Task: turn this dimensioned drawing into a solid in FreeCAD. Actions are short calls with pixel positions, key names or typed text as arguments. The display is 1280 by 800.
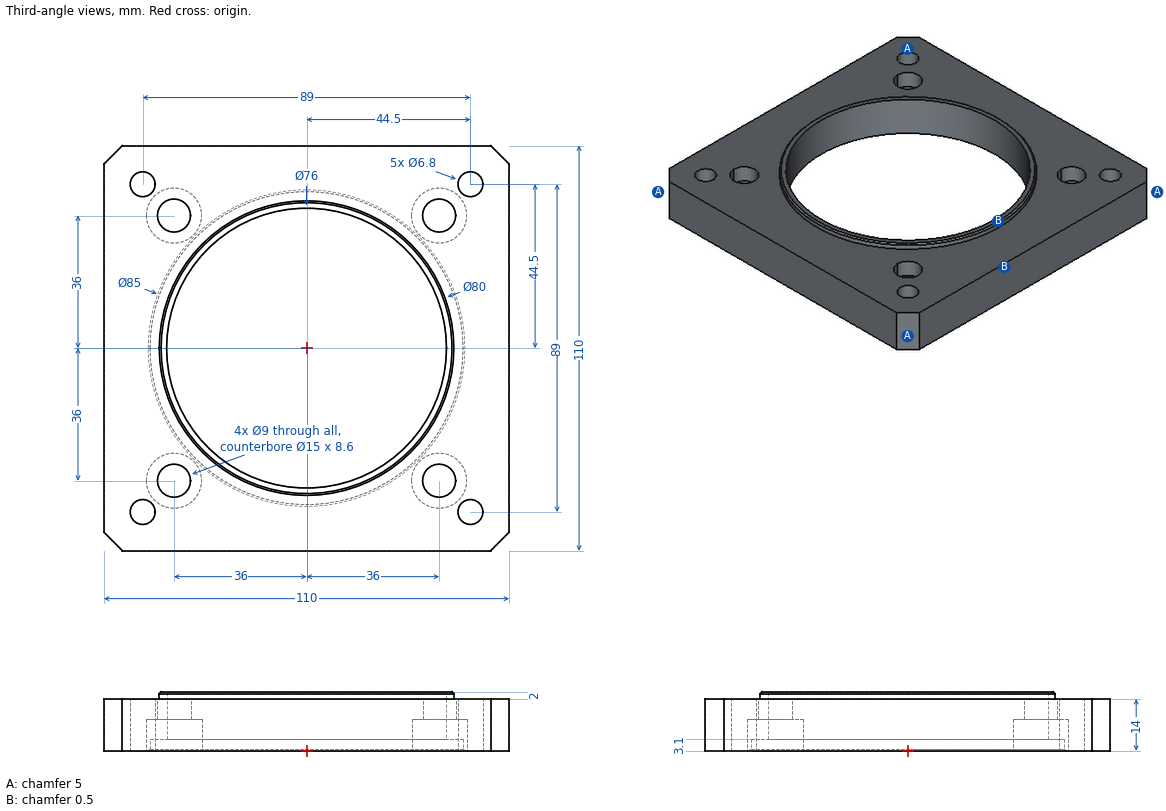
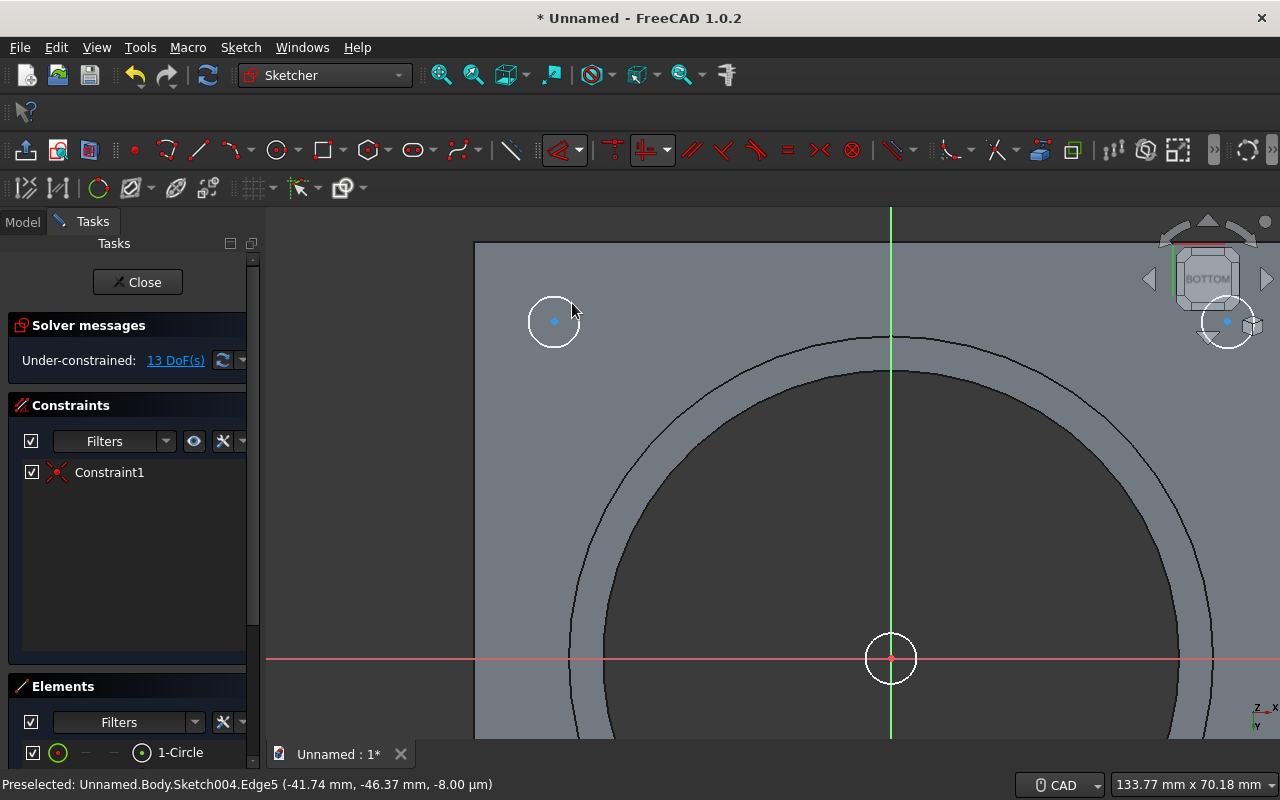
scroll(552, 322, down, 4)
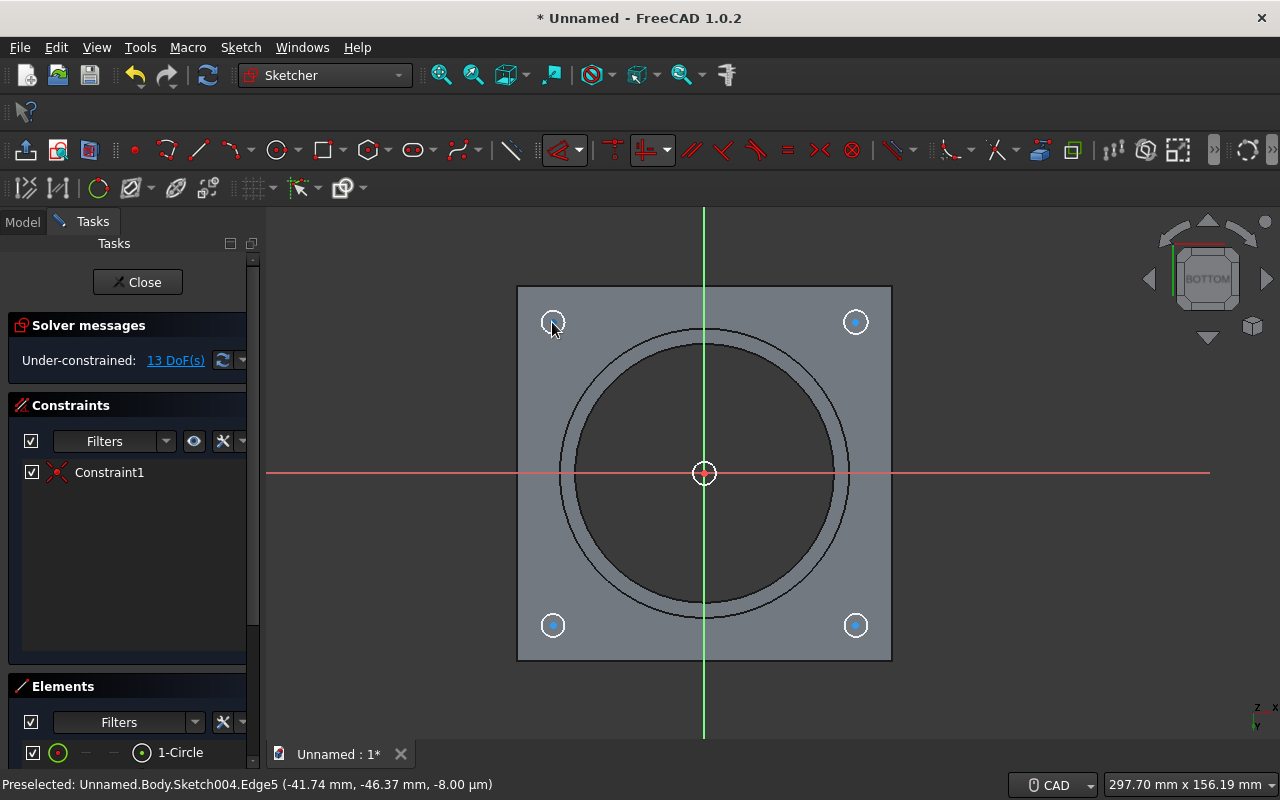
click(864, 617)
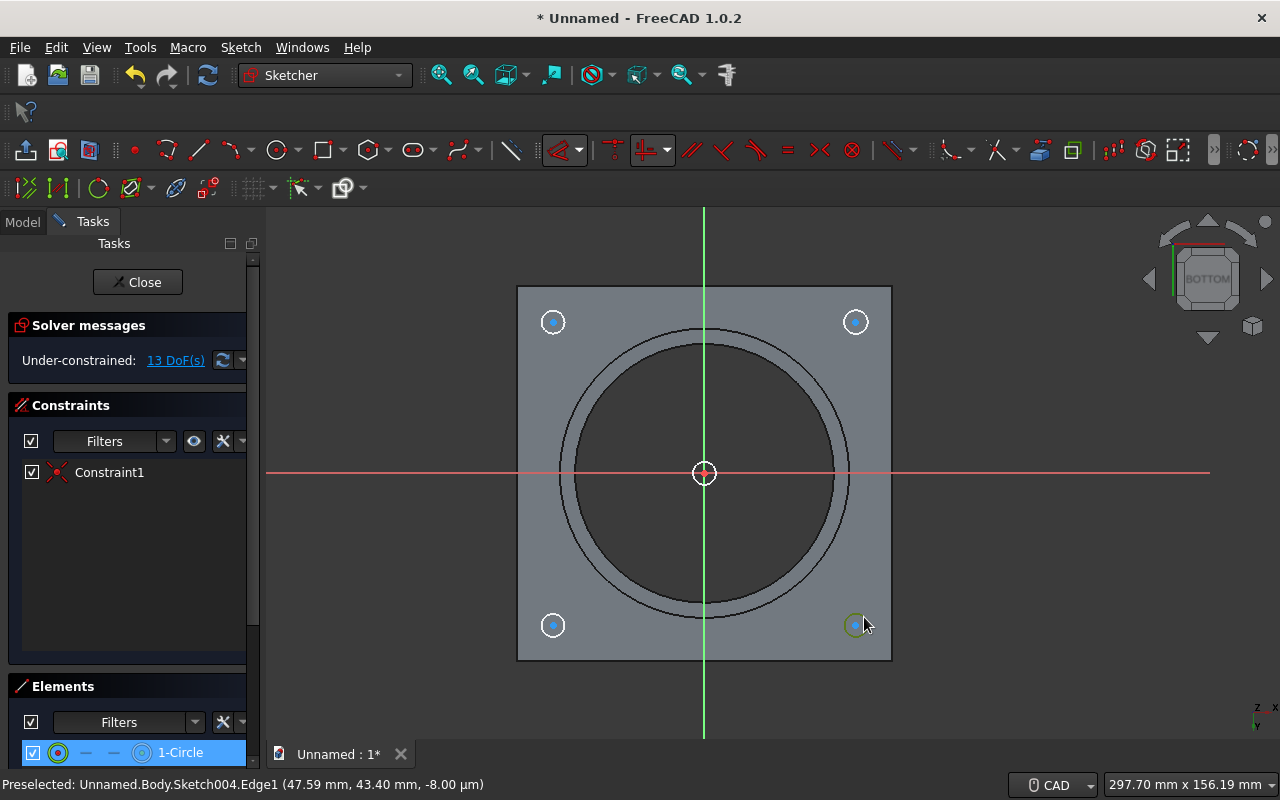
click(705, 462)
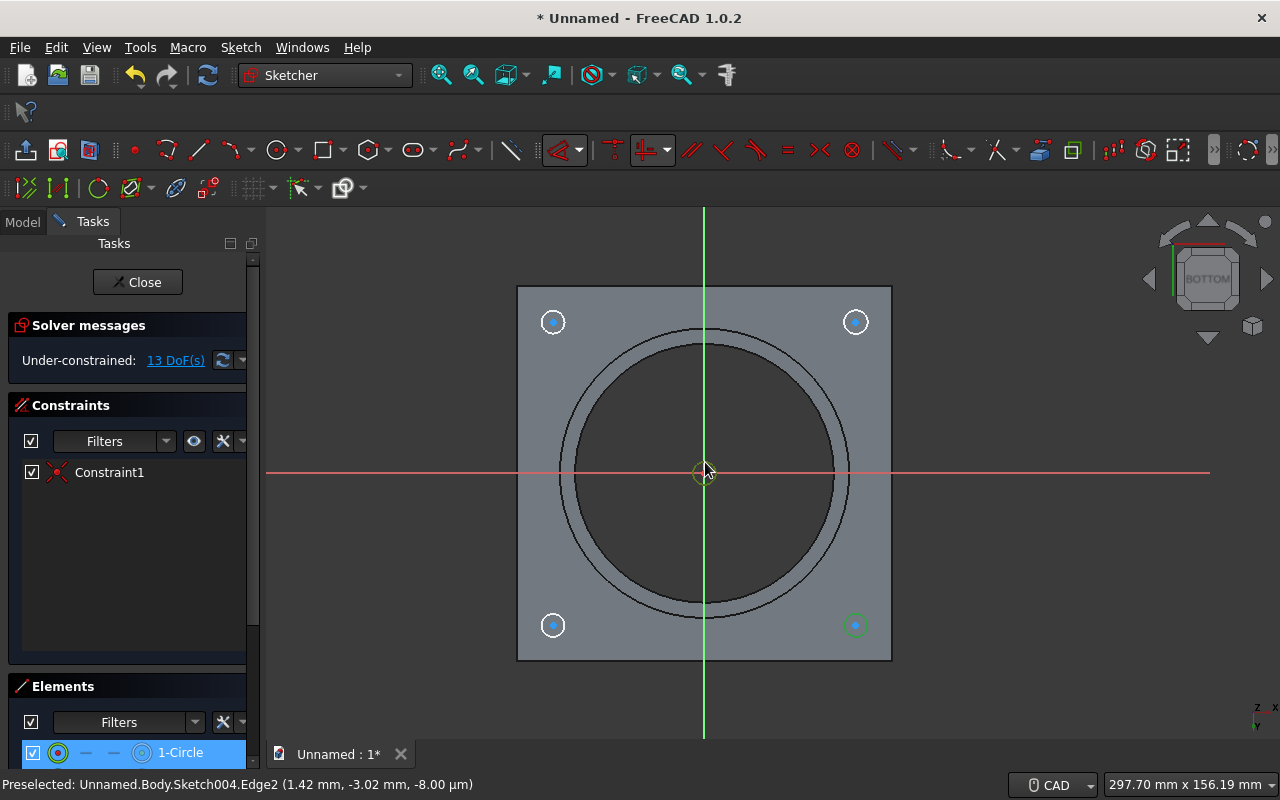
click(561, 617)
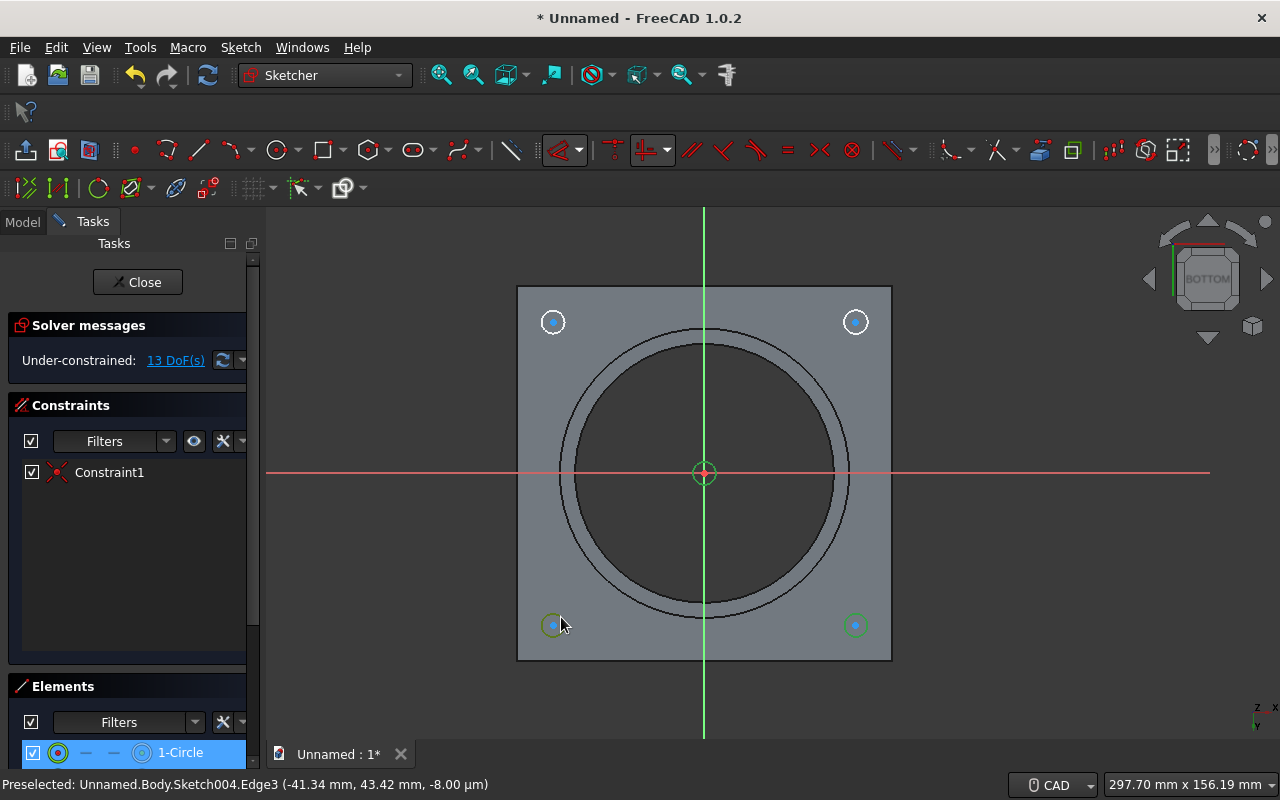
click(864, 314)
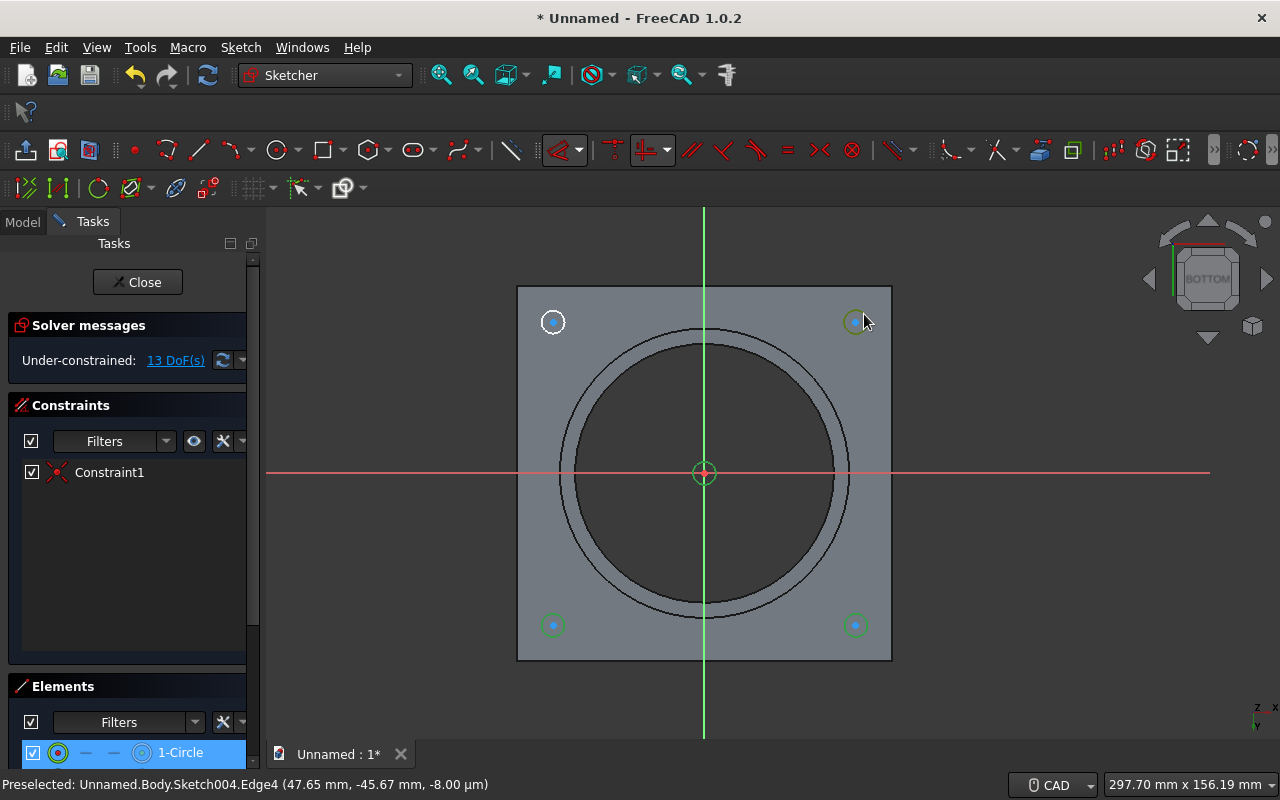
click(561, 314)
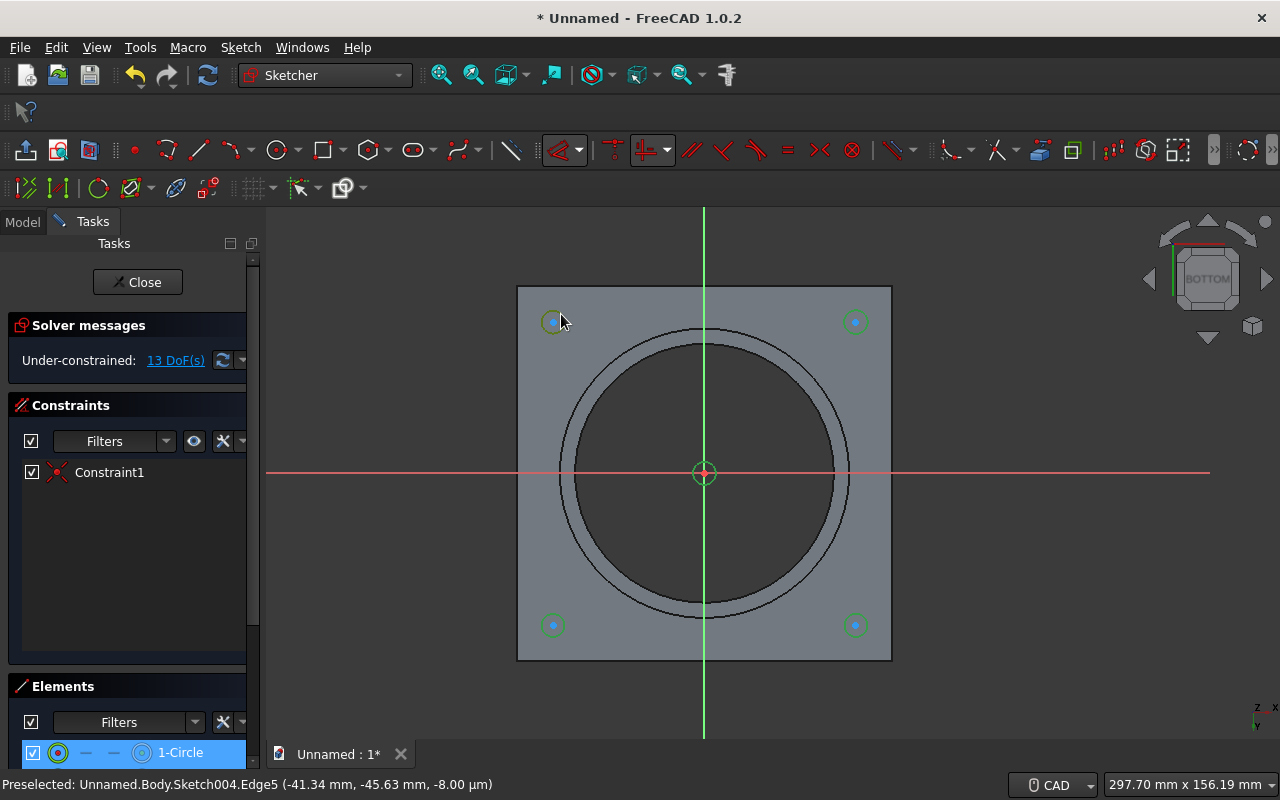
click(788, 150)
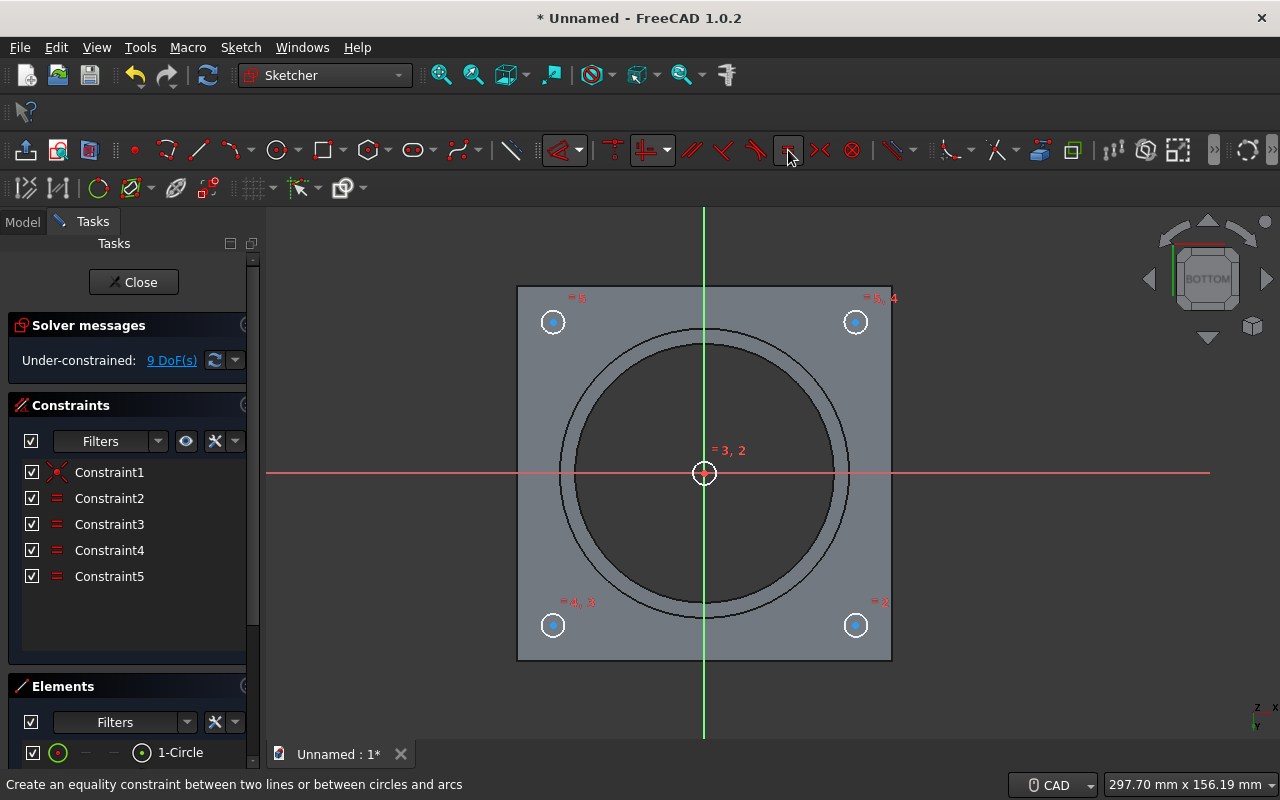
click(856, 625)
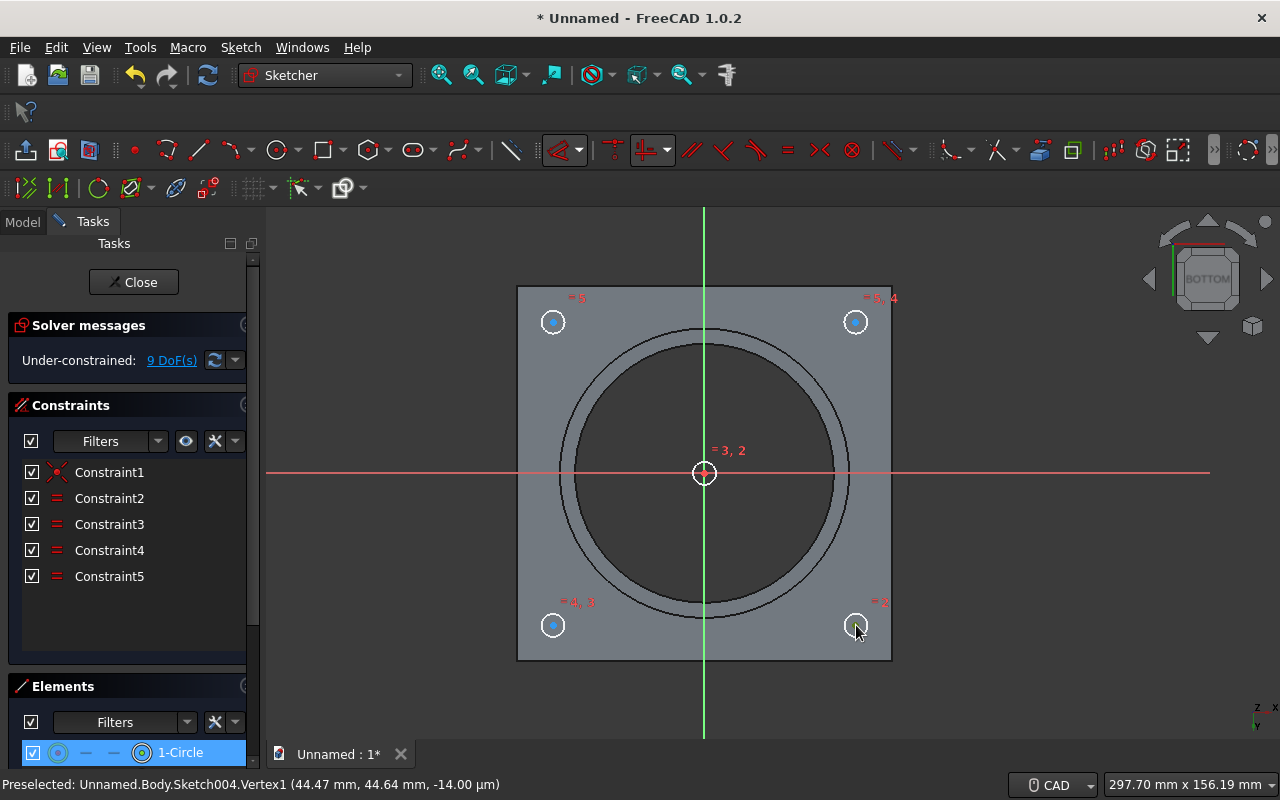
click(553, 625)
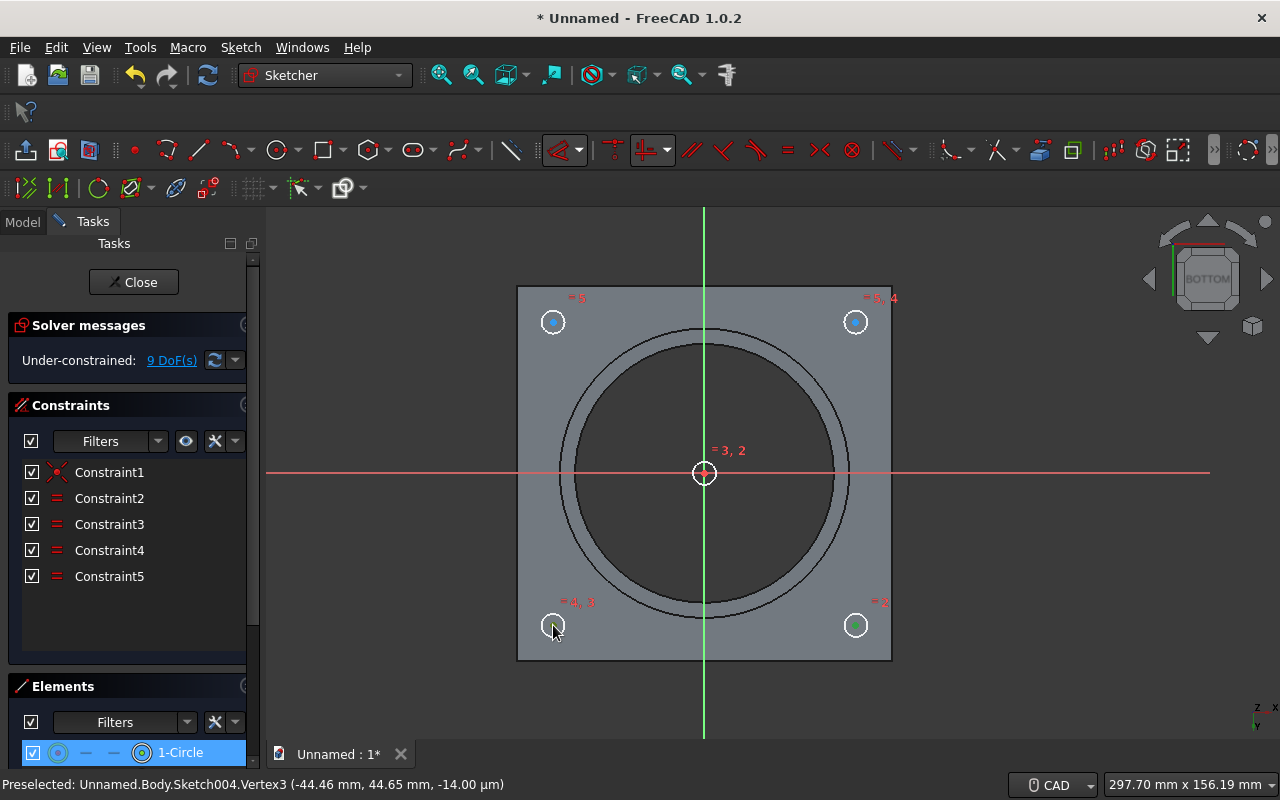
key(h)